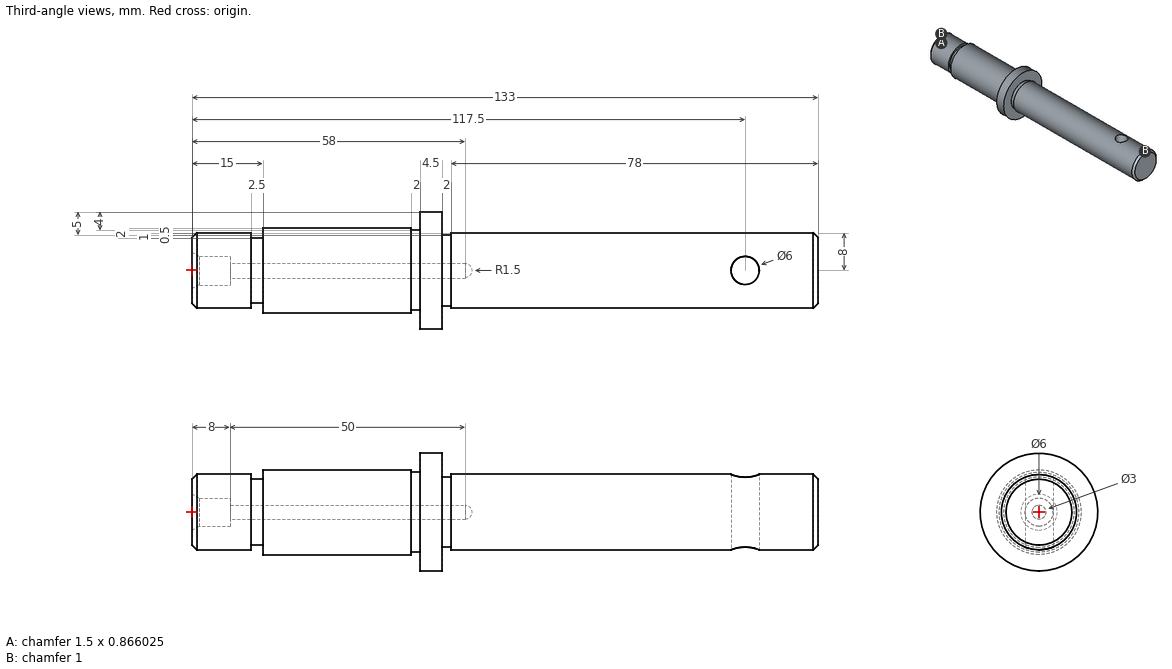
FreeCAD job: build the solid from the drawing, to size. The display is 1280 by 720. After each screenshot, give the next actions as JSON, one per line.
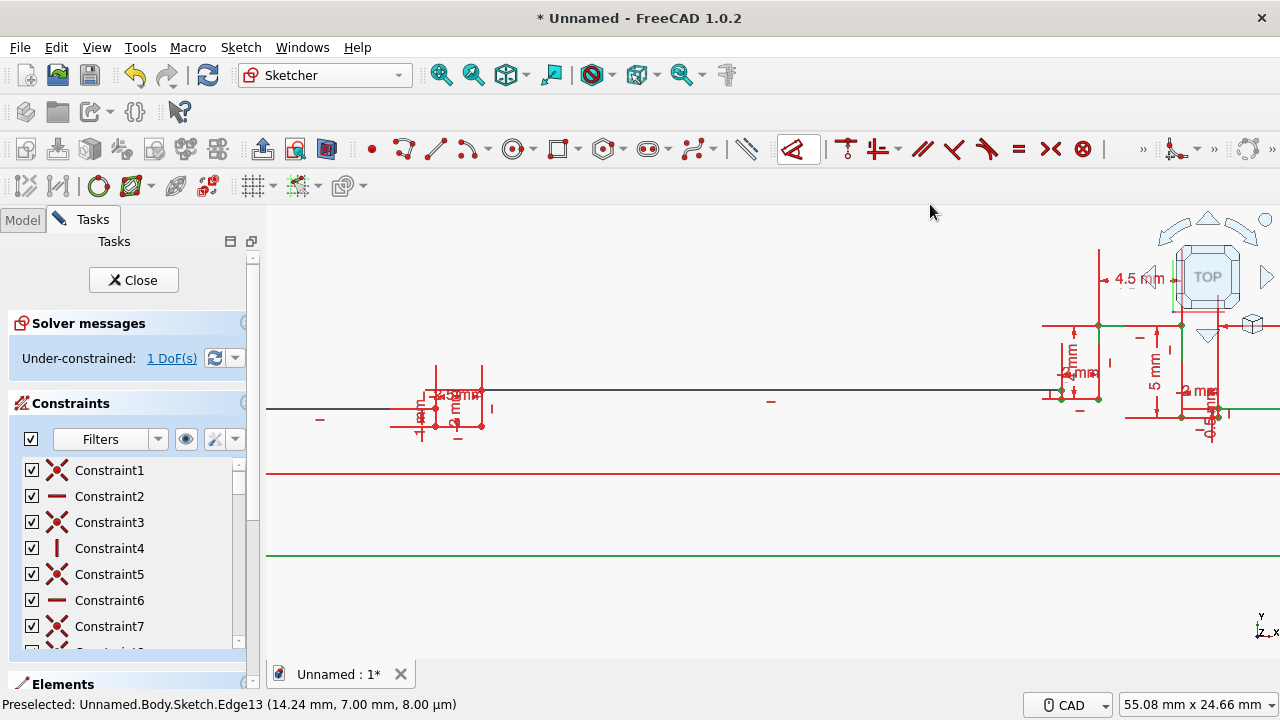
{"action": "scroll", "coordinate": [467, 429], "scroll_direction": "down", "scroll_amount": 7}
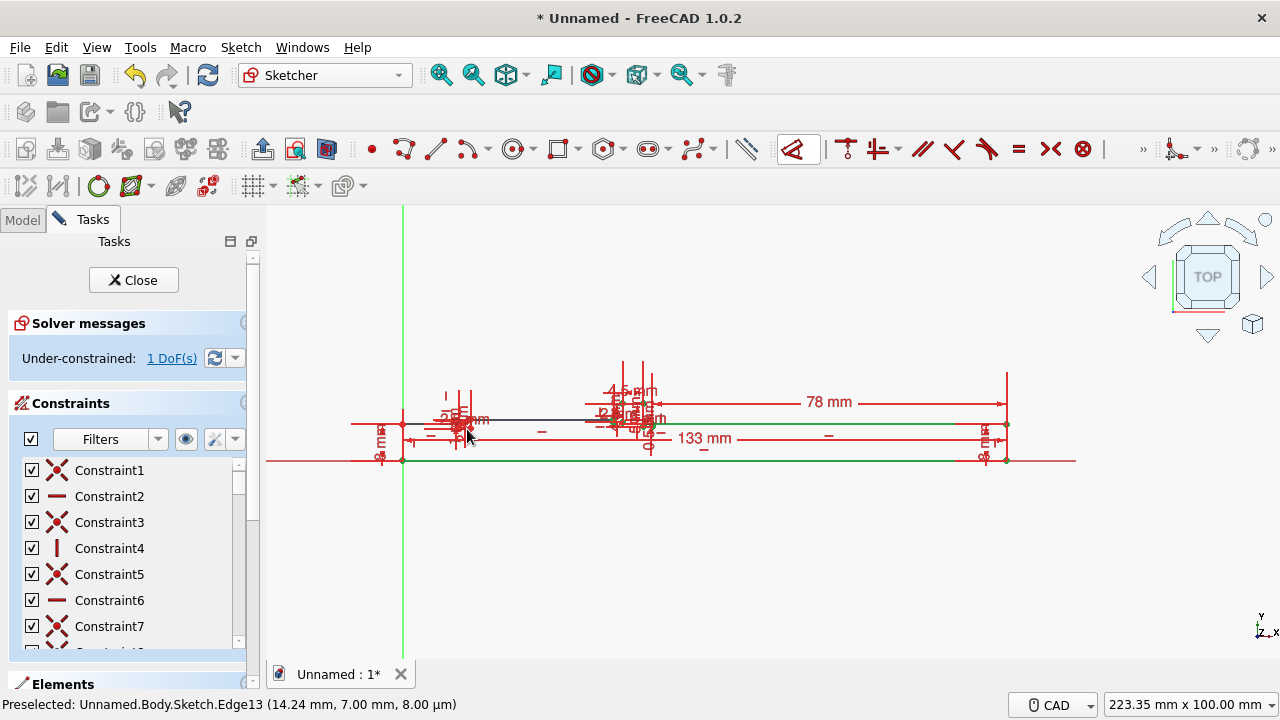
{"action": "scroll", "coordinate": [471, 420], "scroll_direction": "up", "scroll_amount": 2}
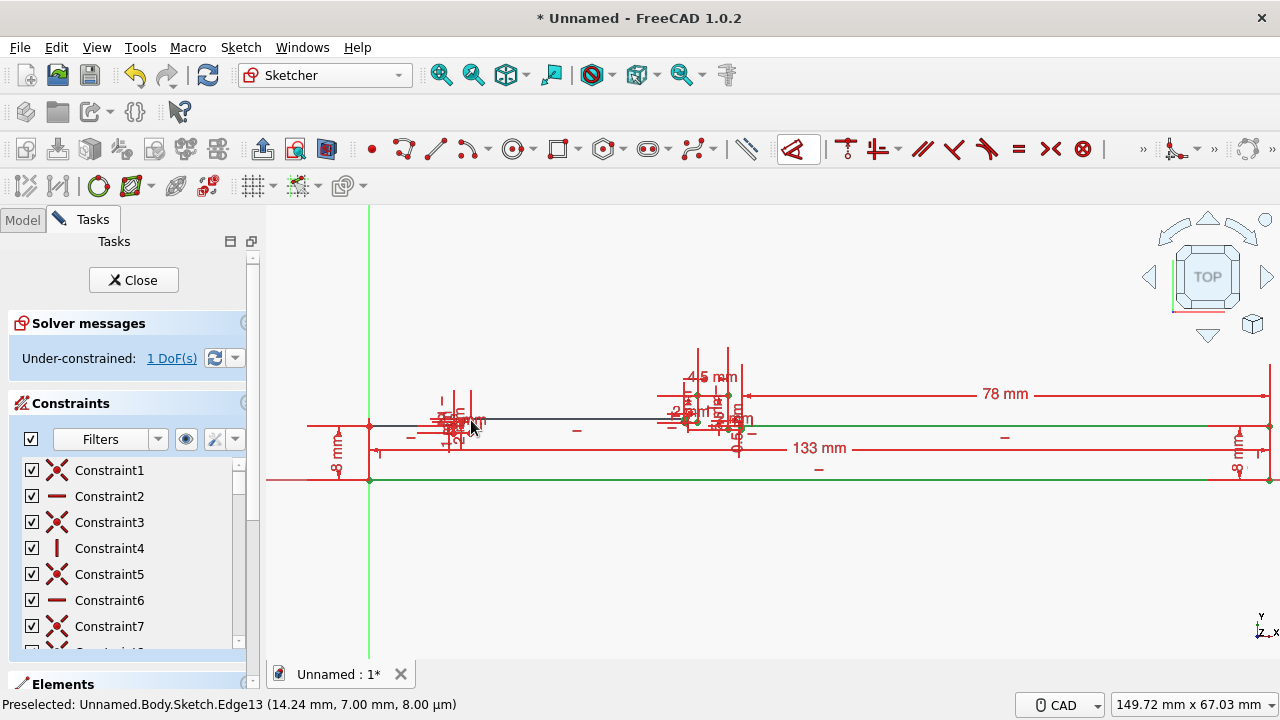
{"action": "left_click", "coordinate": [471, 419]}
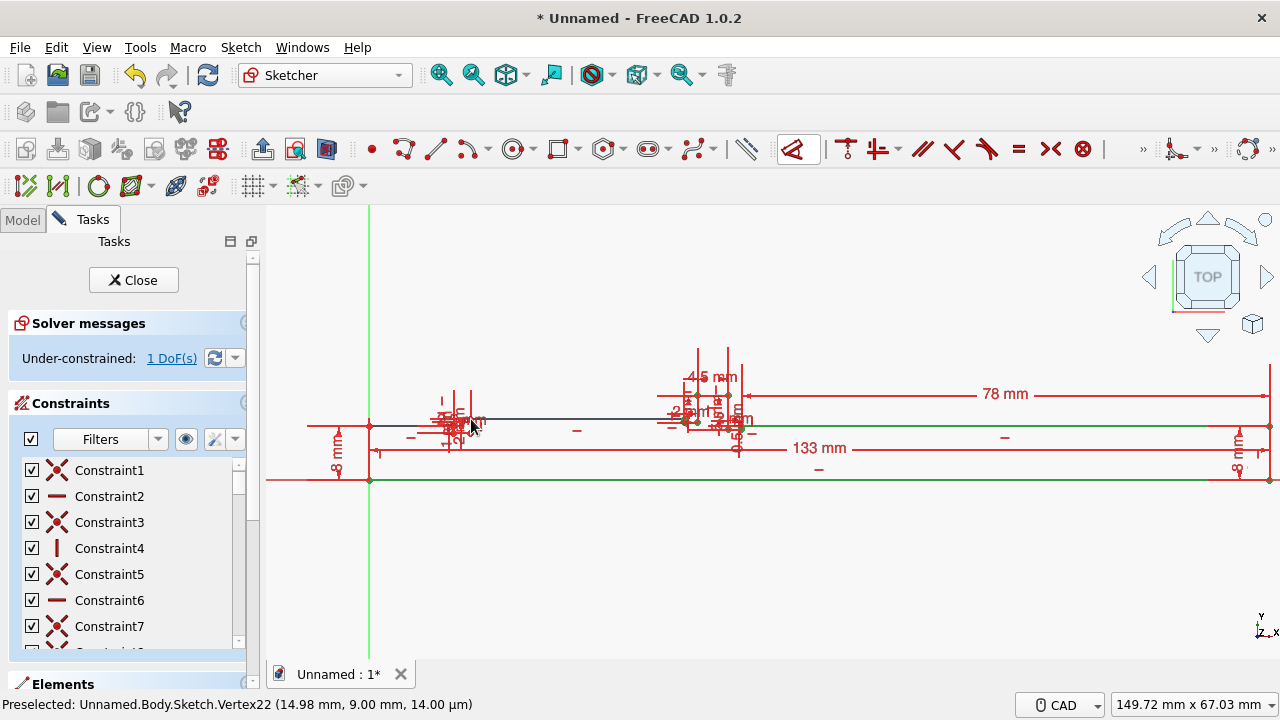
{"action": "key", "text": "l"}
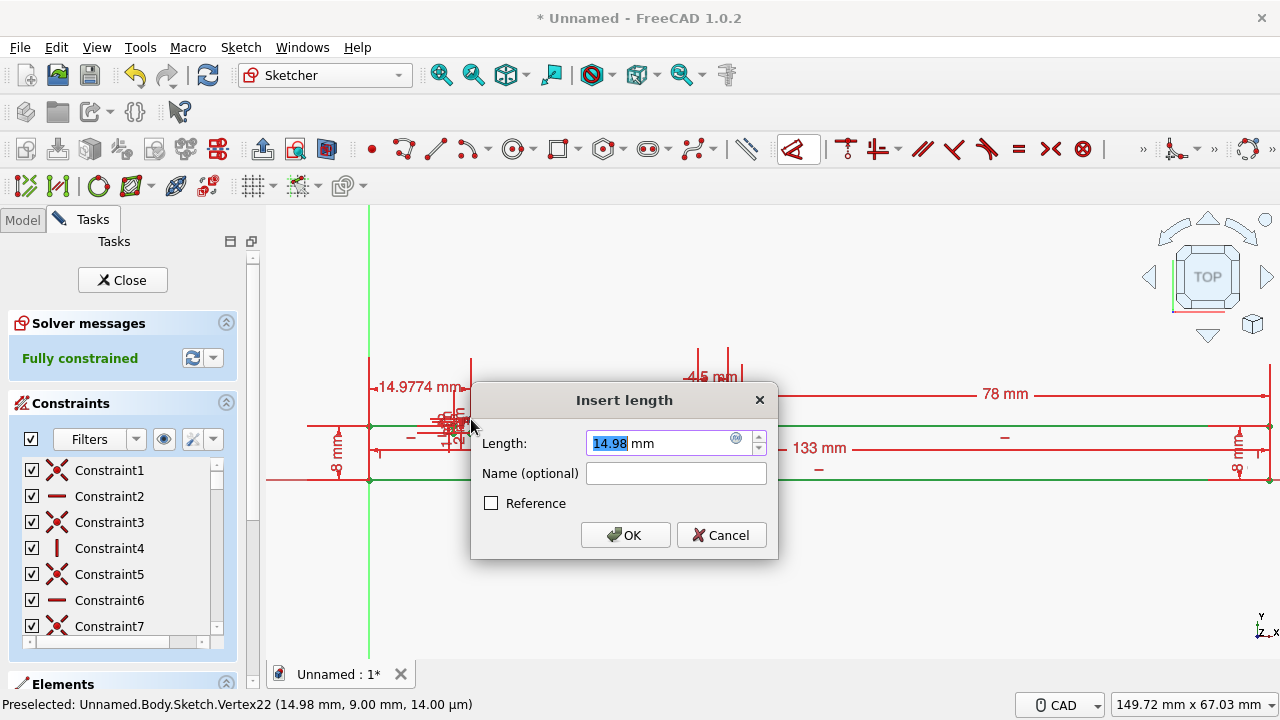
{"action": "type", "text": "15"}
{"action": "key", "text": "Return"}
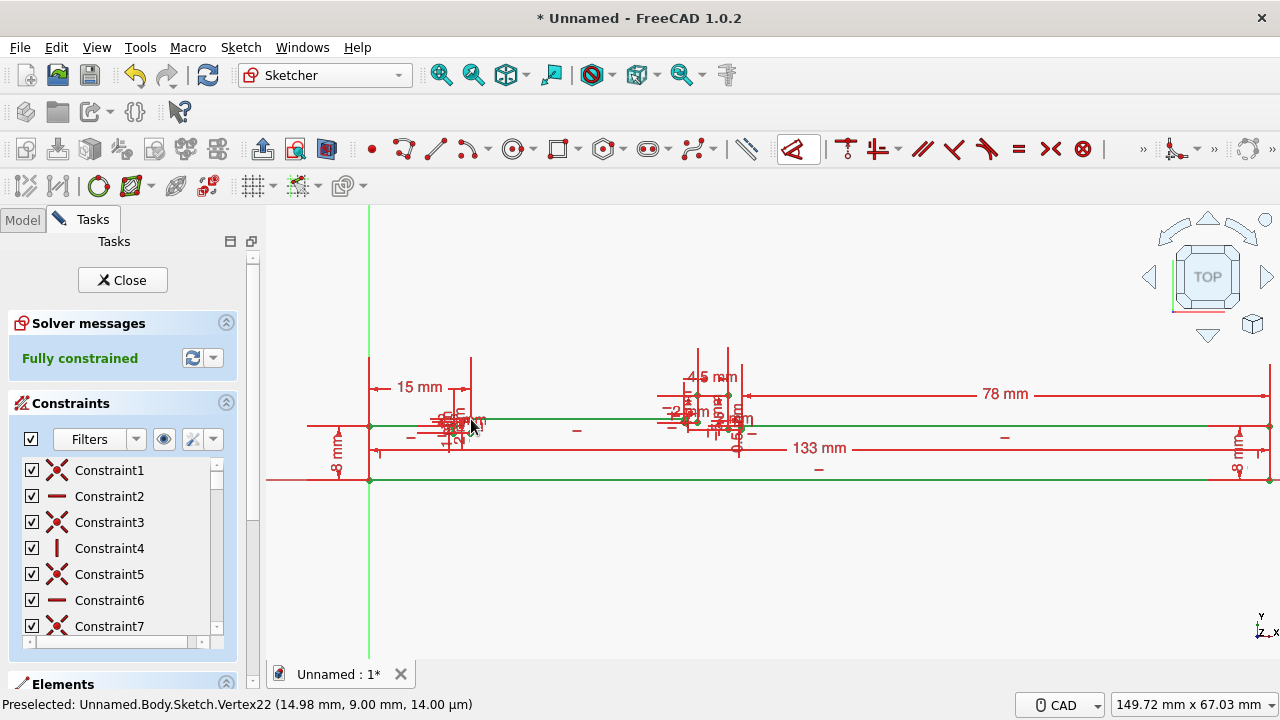
{"action": "left_click", "coordinate": [123, 280]}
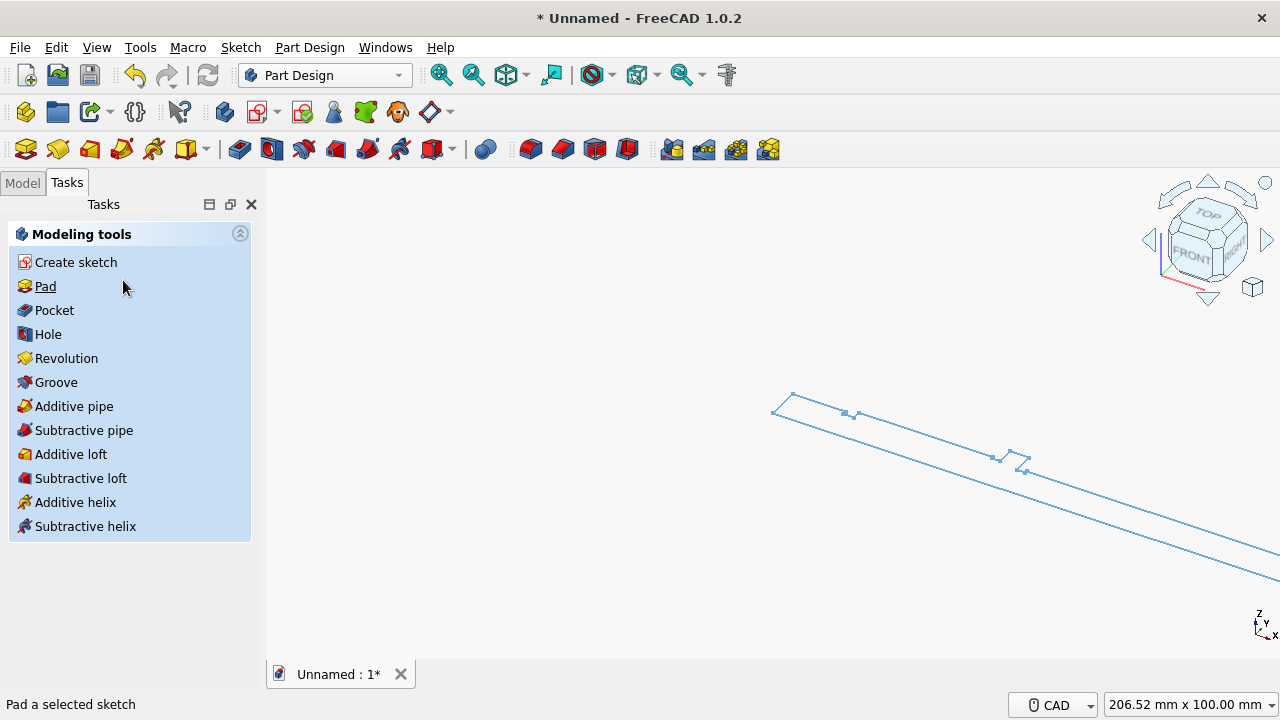
{"action": "left_click", "coordinate": [58, 150]}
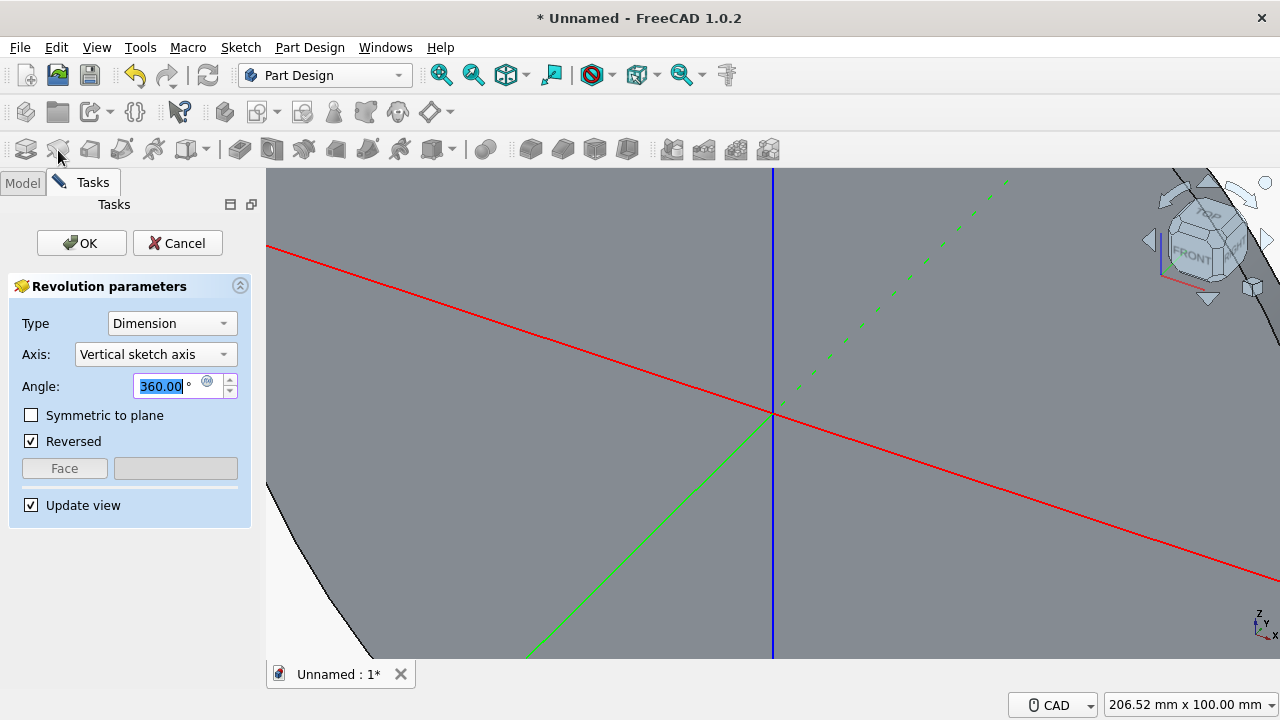
{"action": "left_click", "coordinate": [156, 354]}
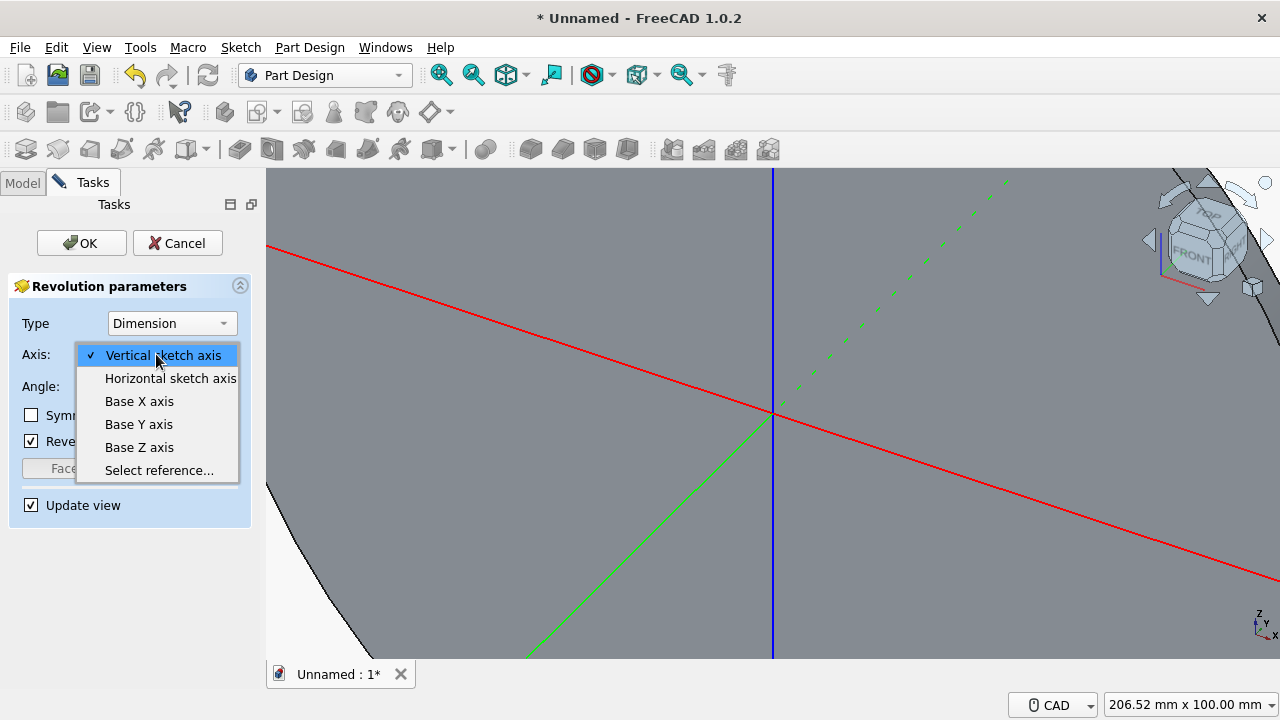
{"action": "left_click", "coordinate": [156, 378]}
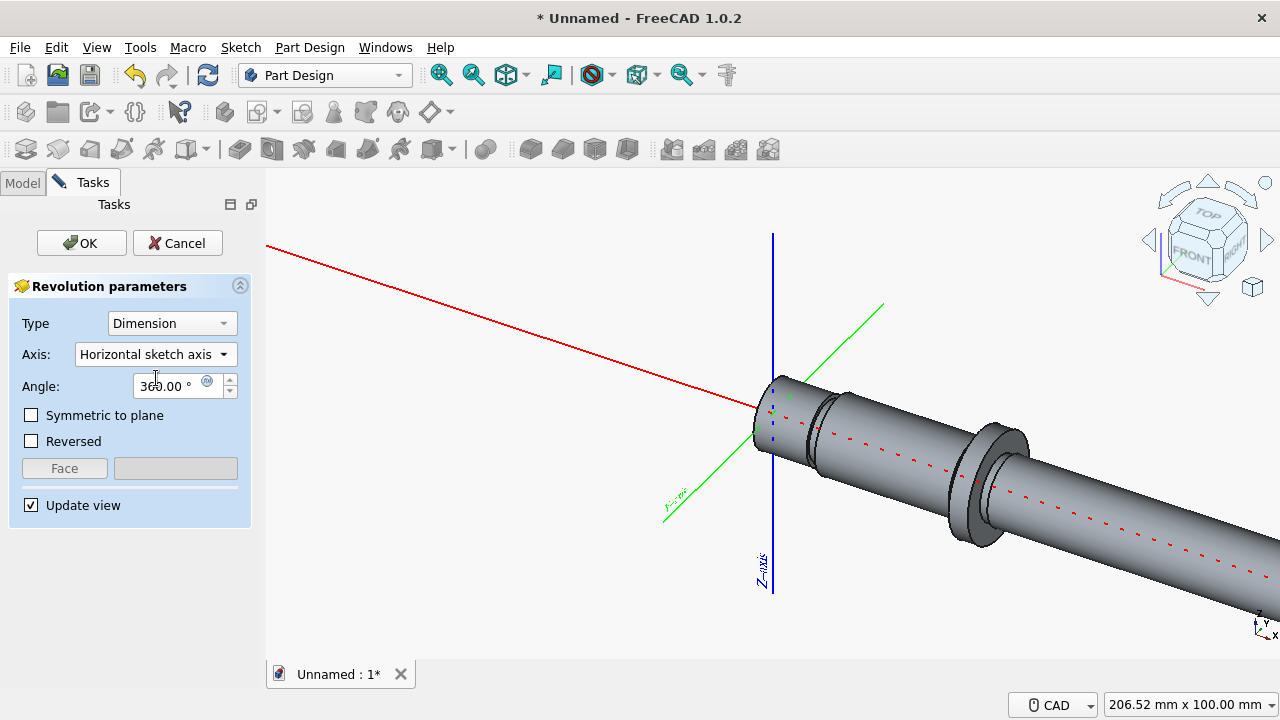
{"action": "left_click", "coordinate": [82, 243]}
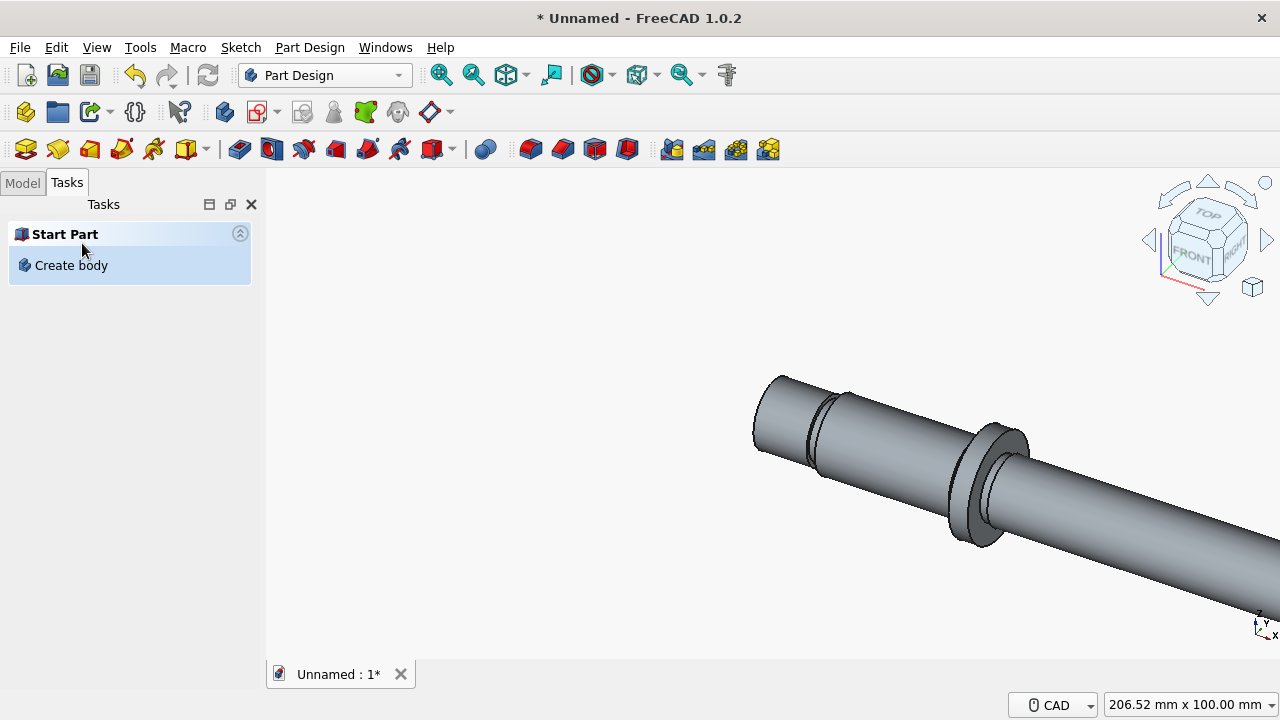
{"action": "left_click", "coordinate": [442, 76]}